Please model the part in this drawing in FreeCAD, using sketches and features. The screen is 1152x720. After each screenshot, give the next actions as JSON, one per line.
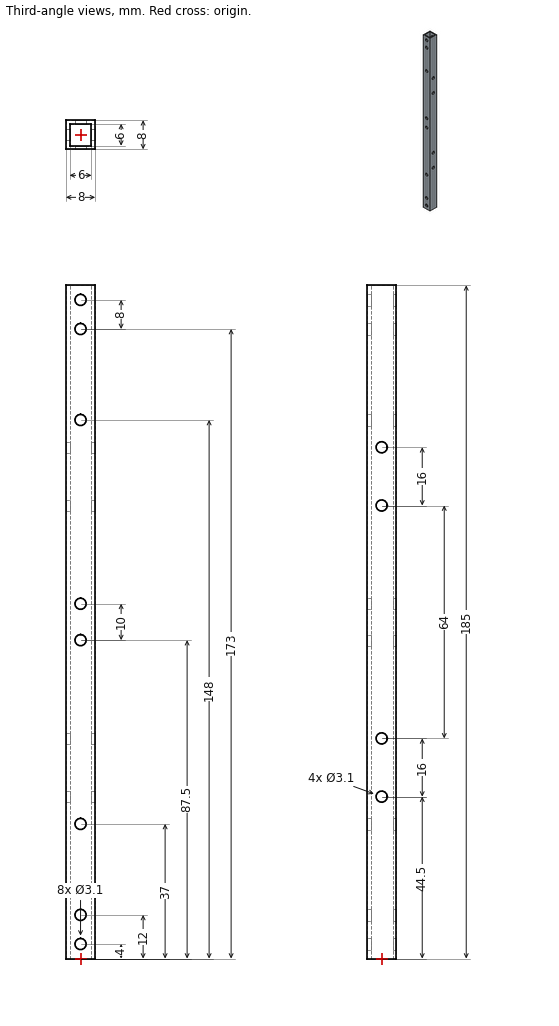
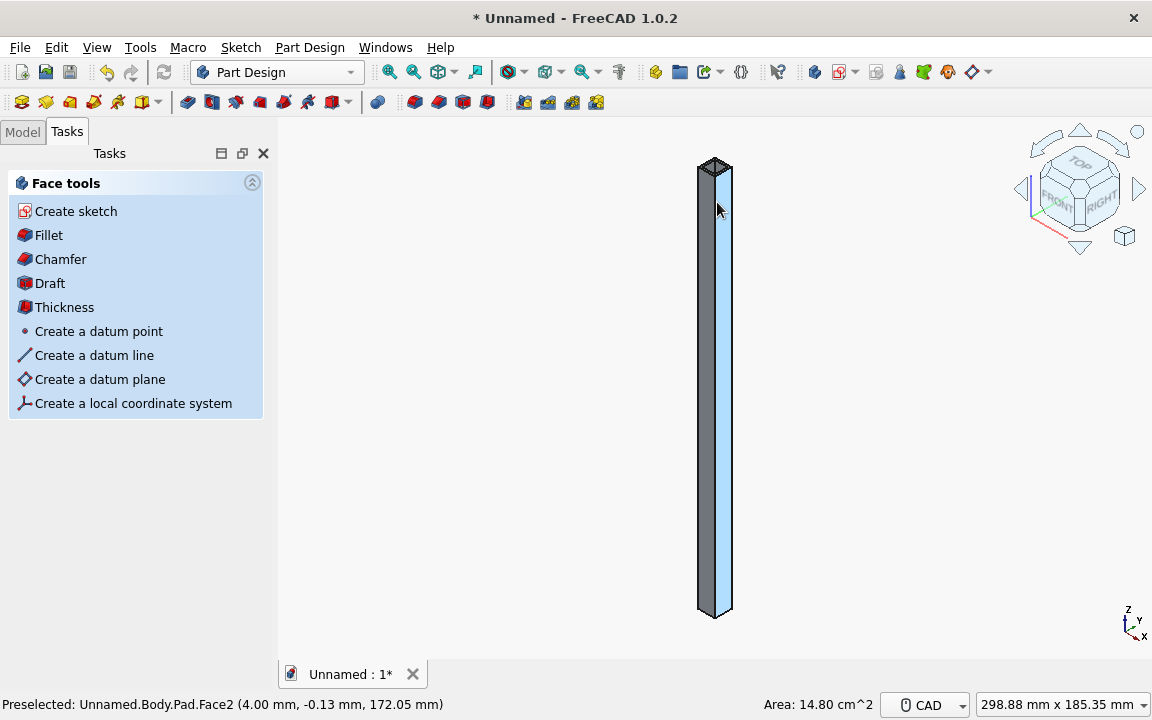
{"action": "left_click", "coordinate": [840, 72]}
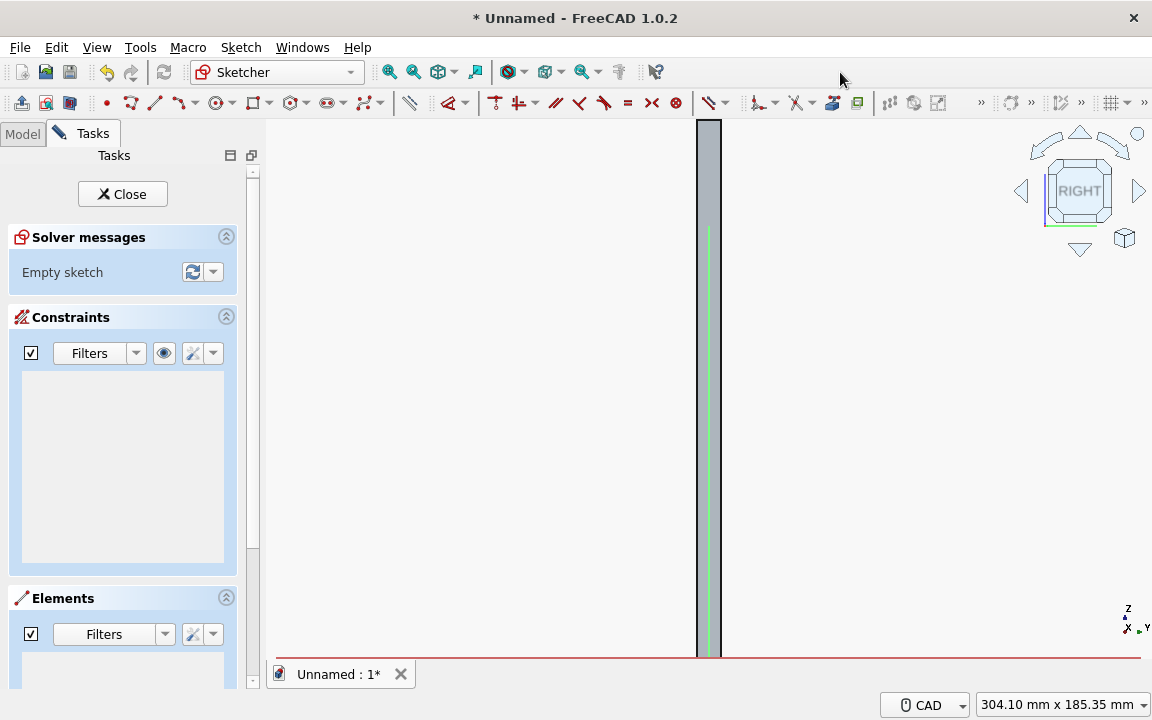
{"action": "scroll", "coordinate": [331, 147], "scroll_direction": "down", "scroll_amount": 1}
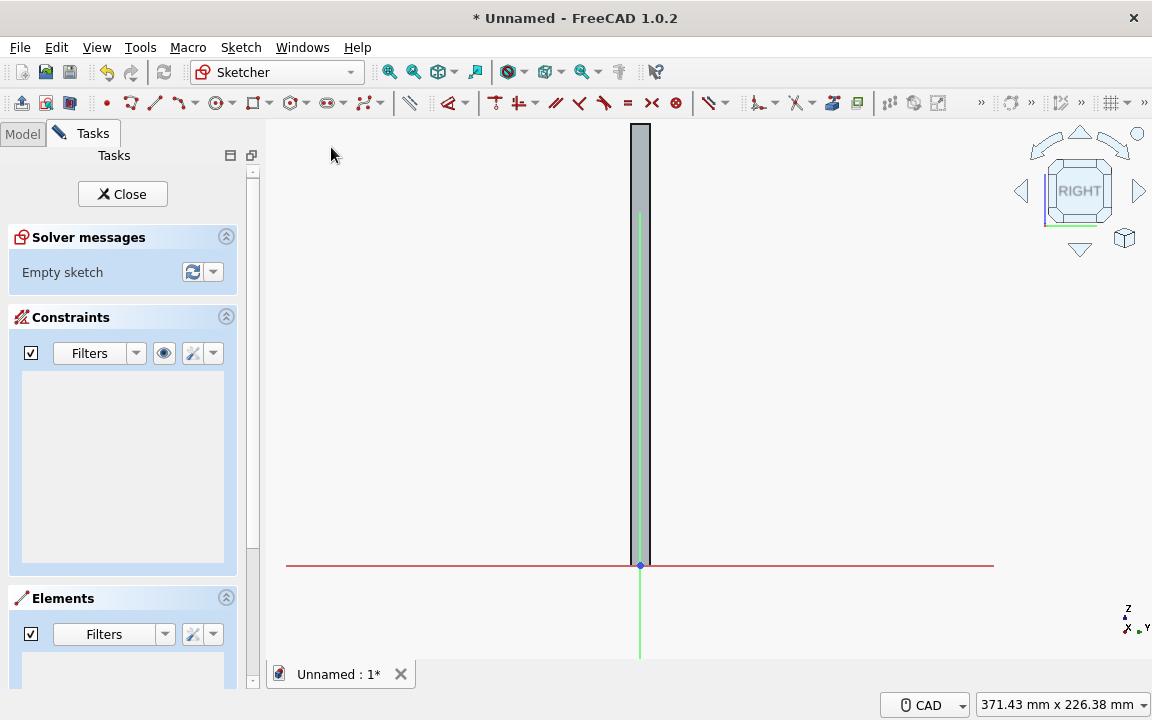
{"action": "left_click", "coordinate": [216, 104]}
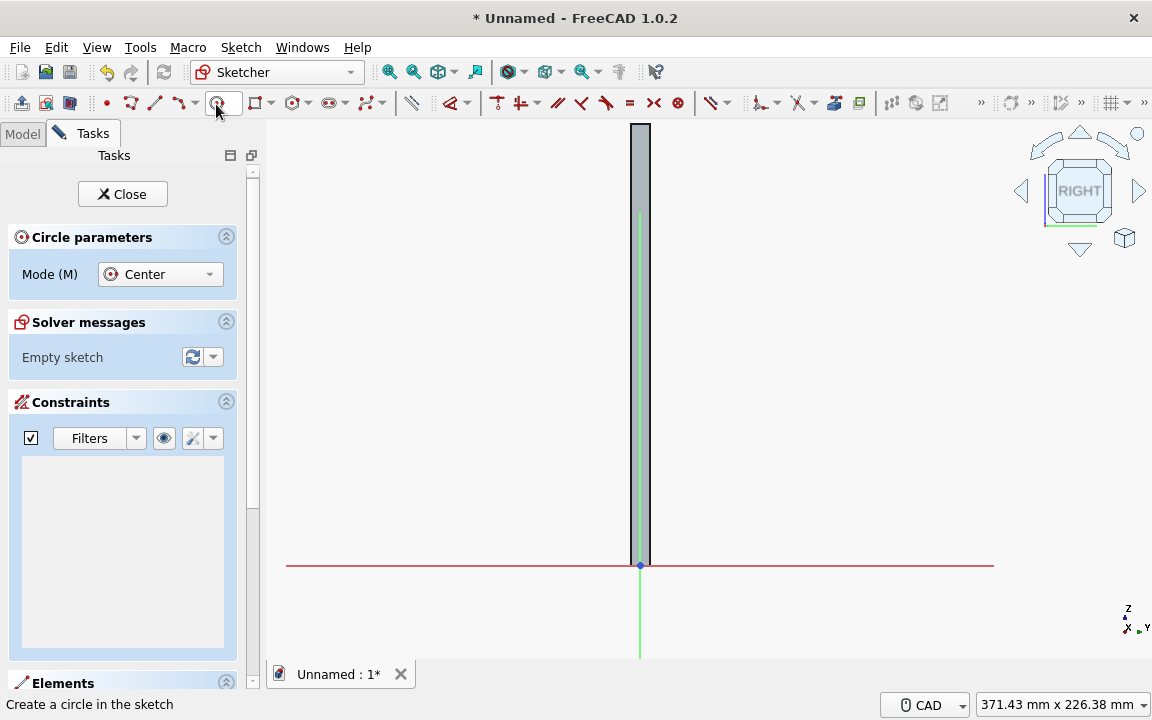
{"action": "scroll", "coordinate": [640, 460], "scroll_direction": "up", "scroll_amount": 10}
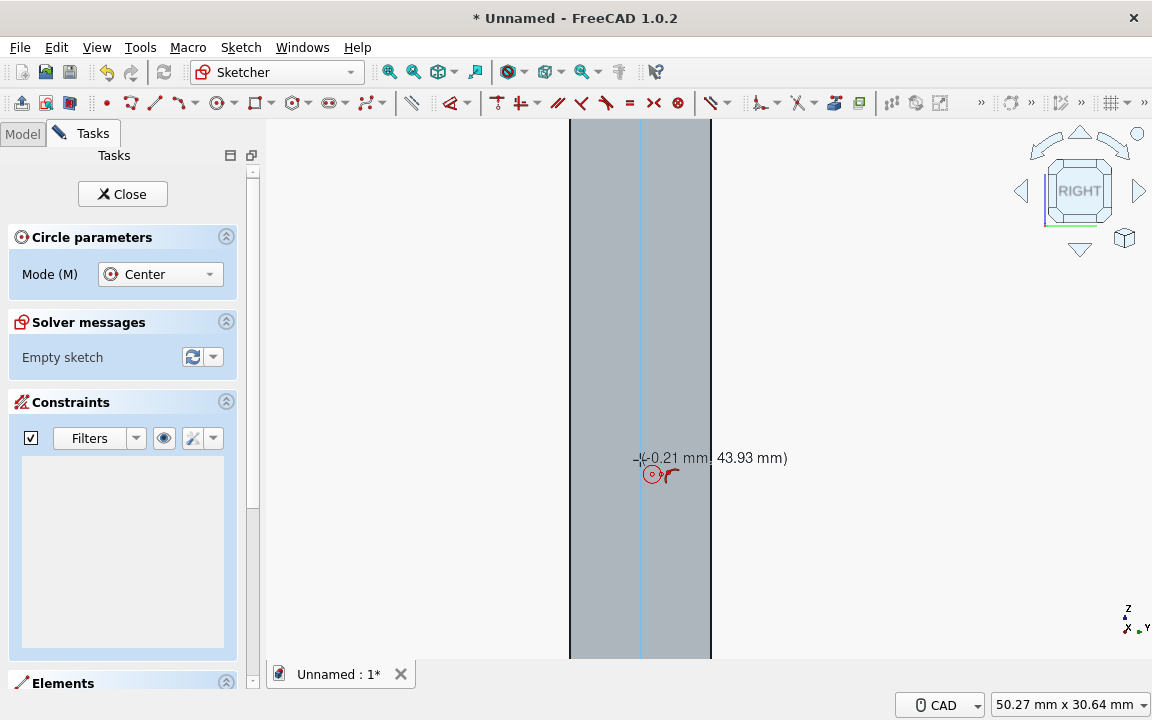
{"action": "scroll", "coordinate": [640, 452], "scroll_direction": "down", "scroll_amount": 10}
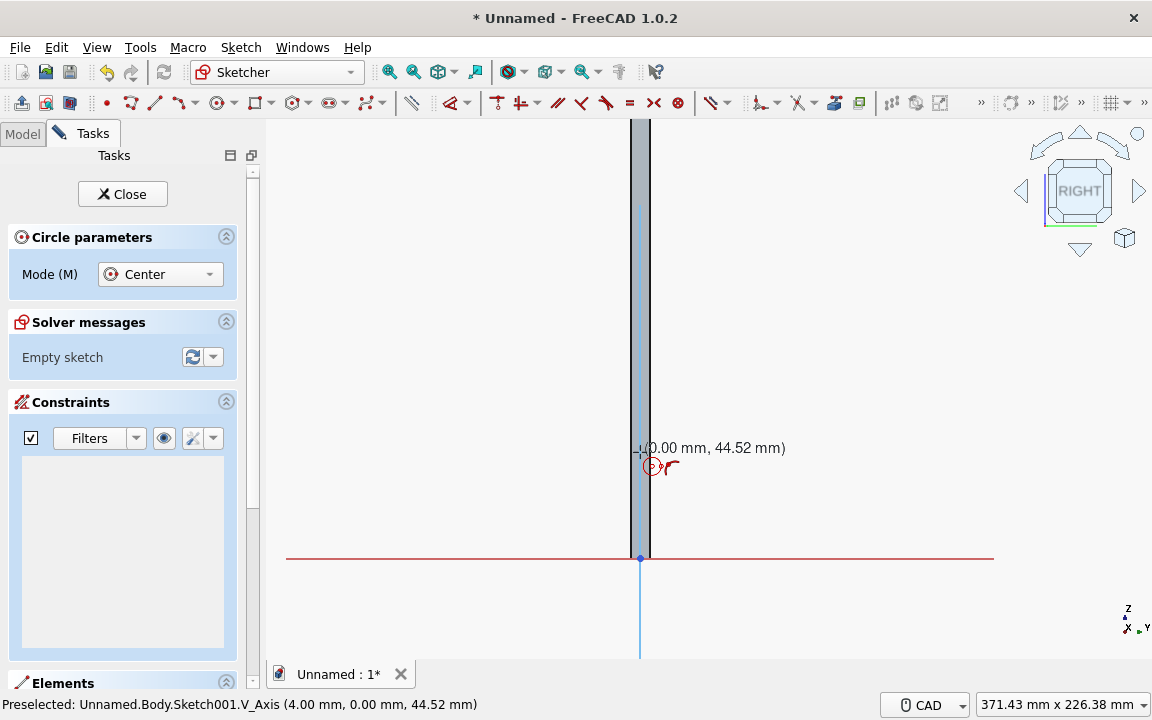
{"action": "left_click", "coordinate": [640, 453]}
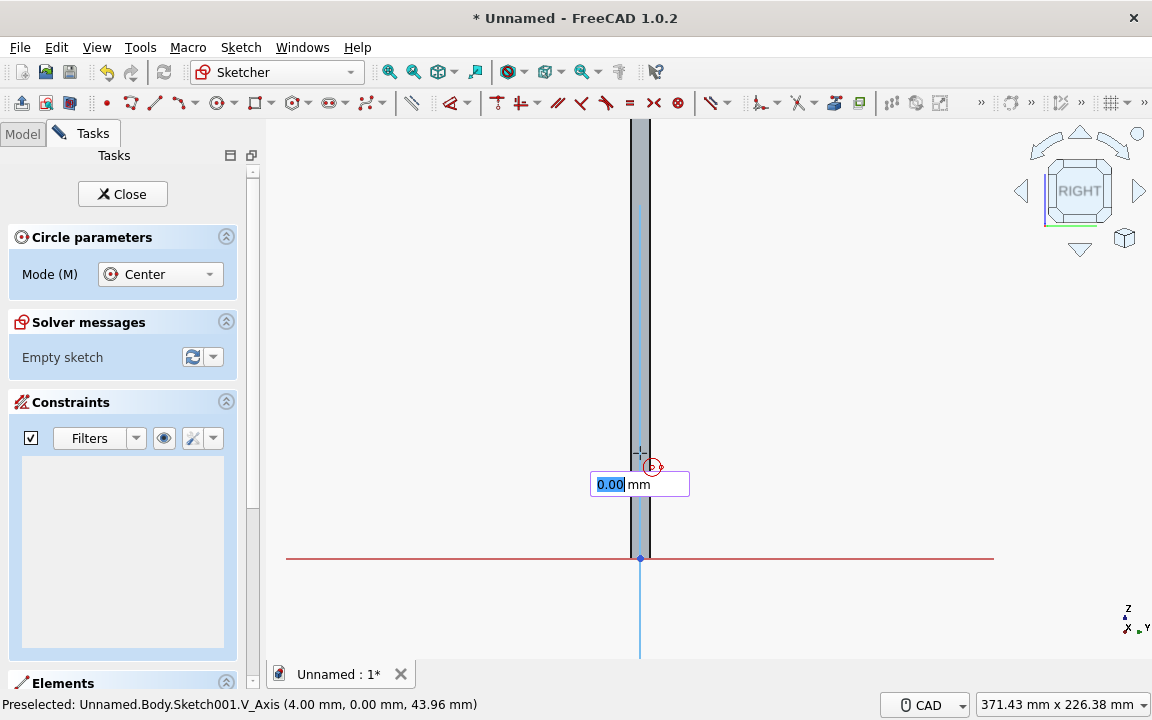
{"action": "scroll", "coordinate": [644, 451], "scroll_direction": "up", "scroll_amount": 8}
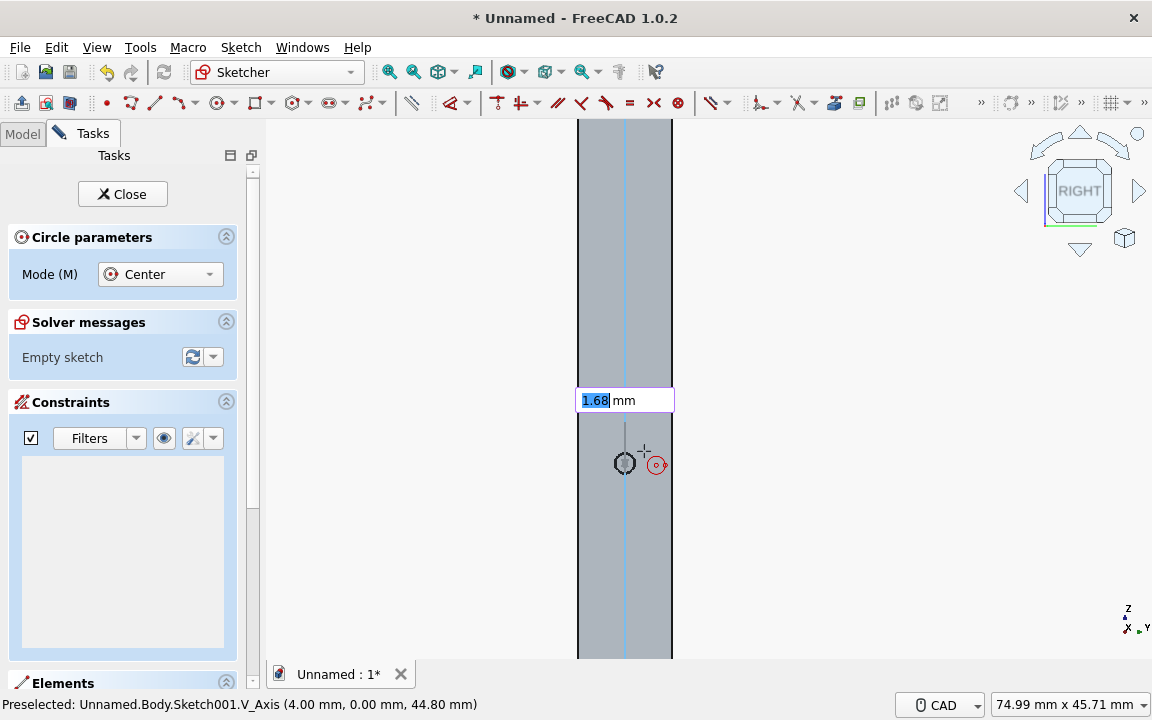
{"action": "left_click", "coordinate": [642, 451]}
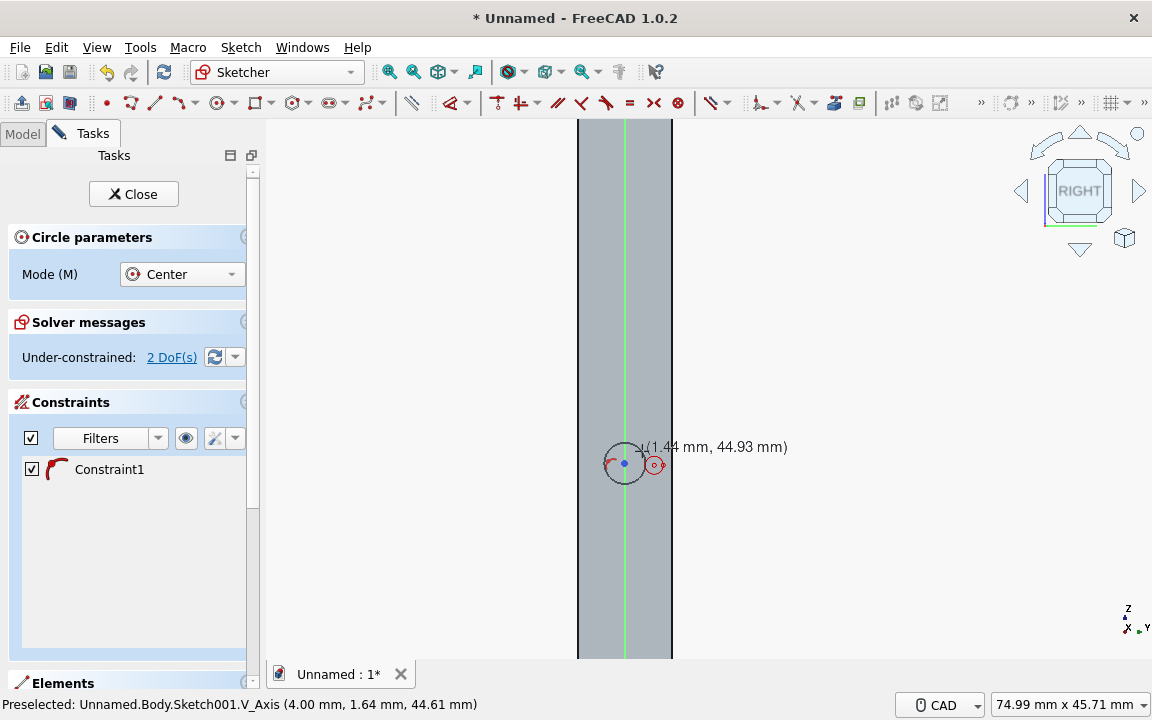
{"action": "scroll", "coordinate": [625, 268], "scroll_direction": "up", "scroll_amount": 2}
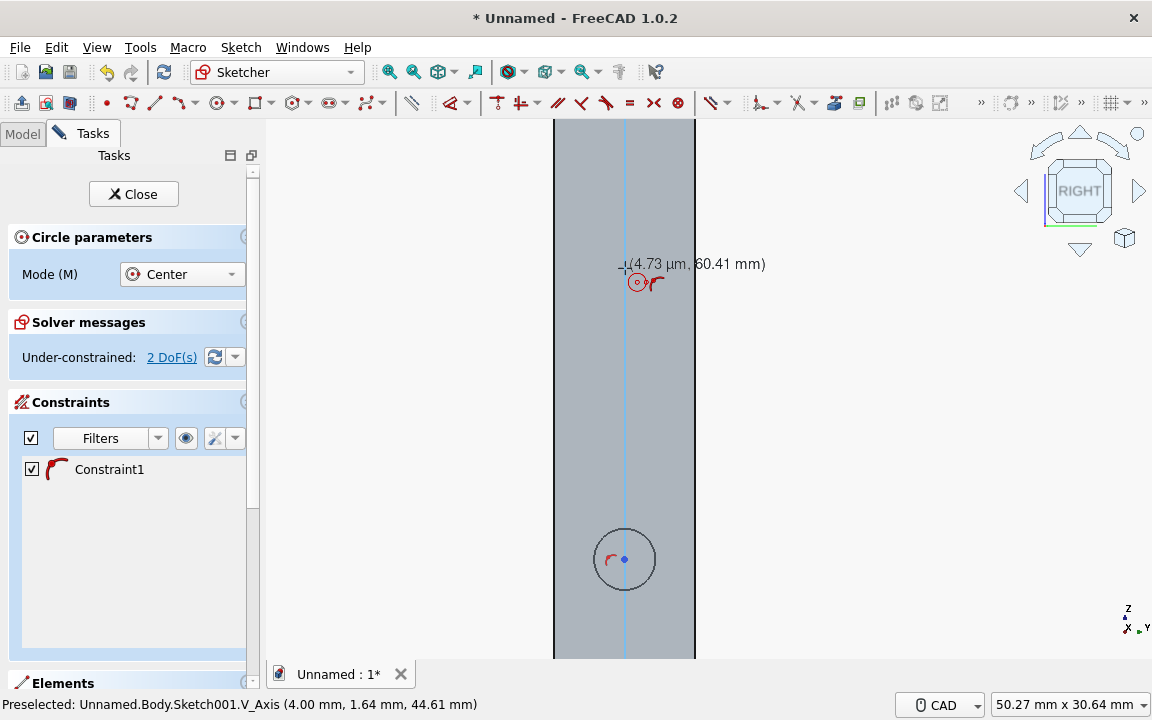
{"action": "scroll", "coordinate": [643, 437], "scroll_direction": "down", "scroll_amount": 10}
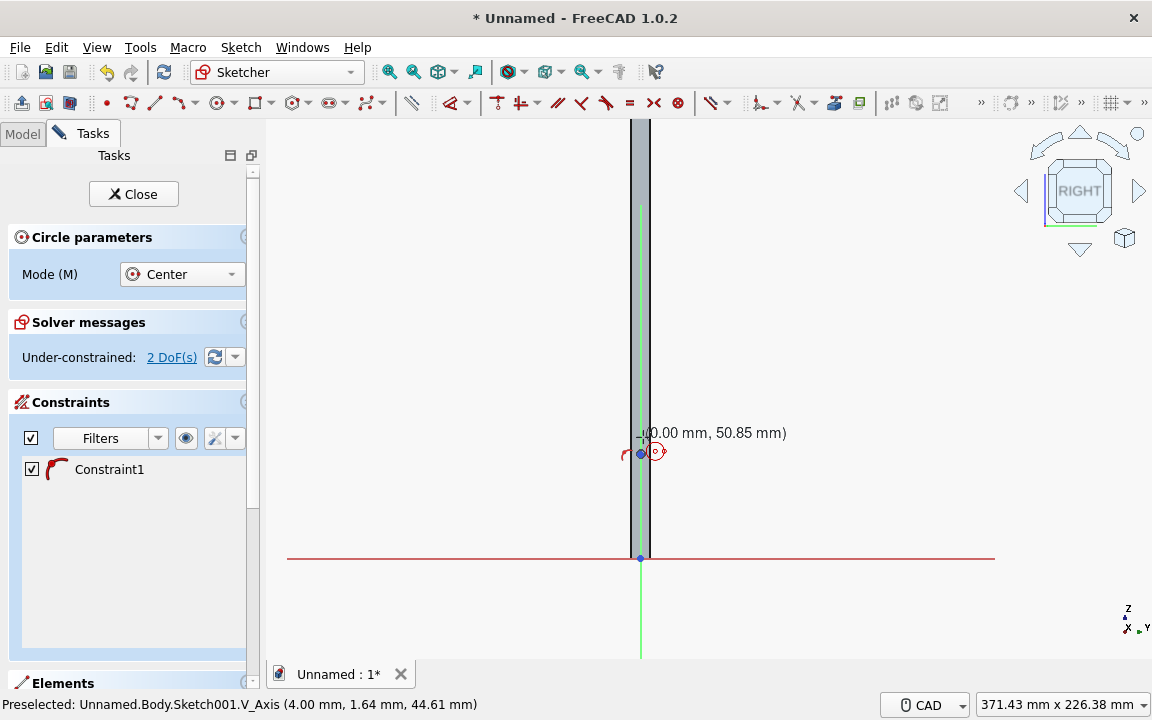
{"action": "left_click", "coordinate": [641, 415]}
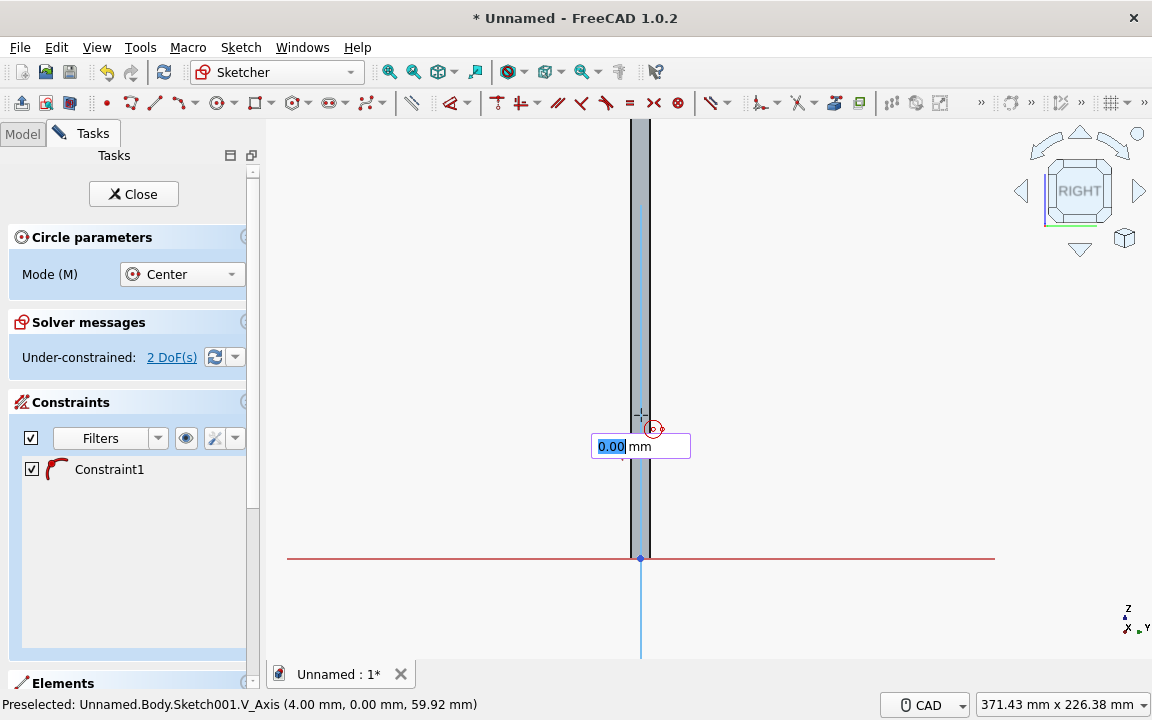
{"action": "scroll", "coordinate": [644, 413], "scroll_direction": "up", "scroll_amount": 8}